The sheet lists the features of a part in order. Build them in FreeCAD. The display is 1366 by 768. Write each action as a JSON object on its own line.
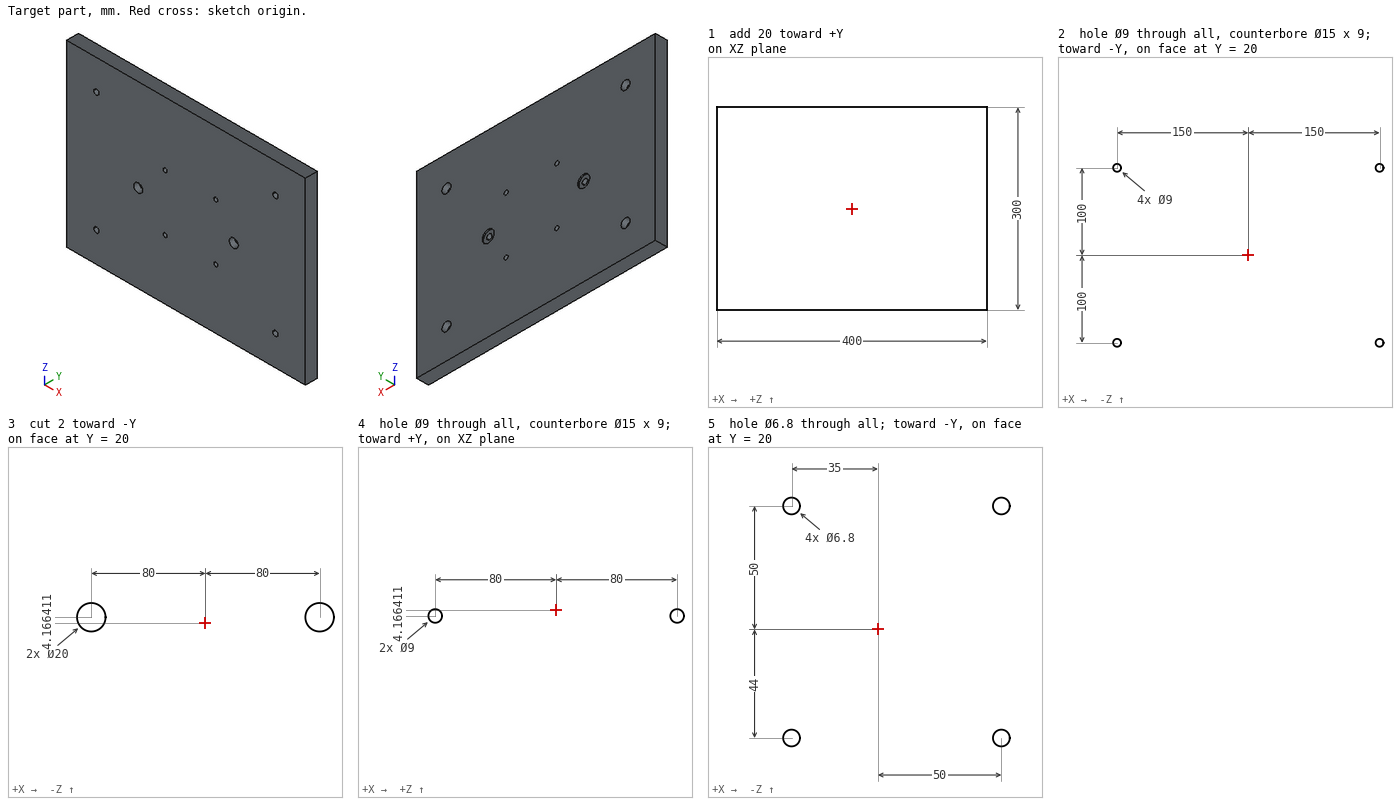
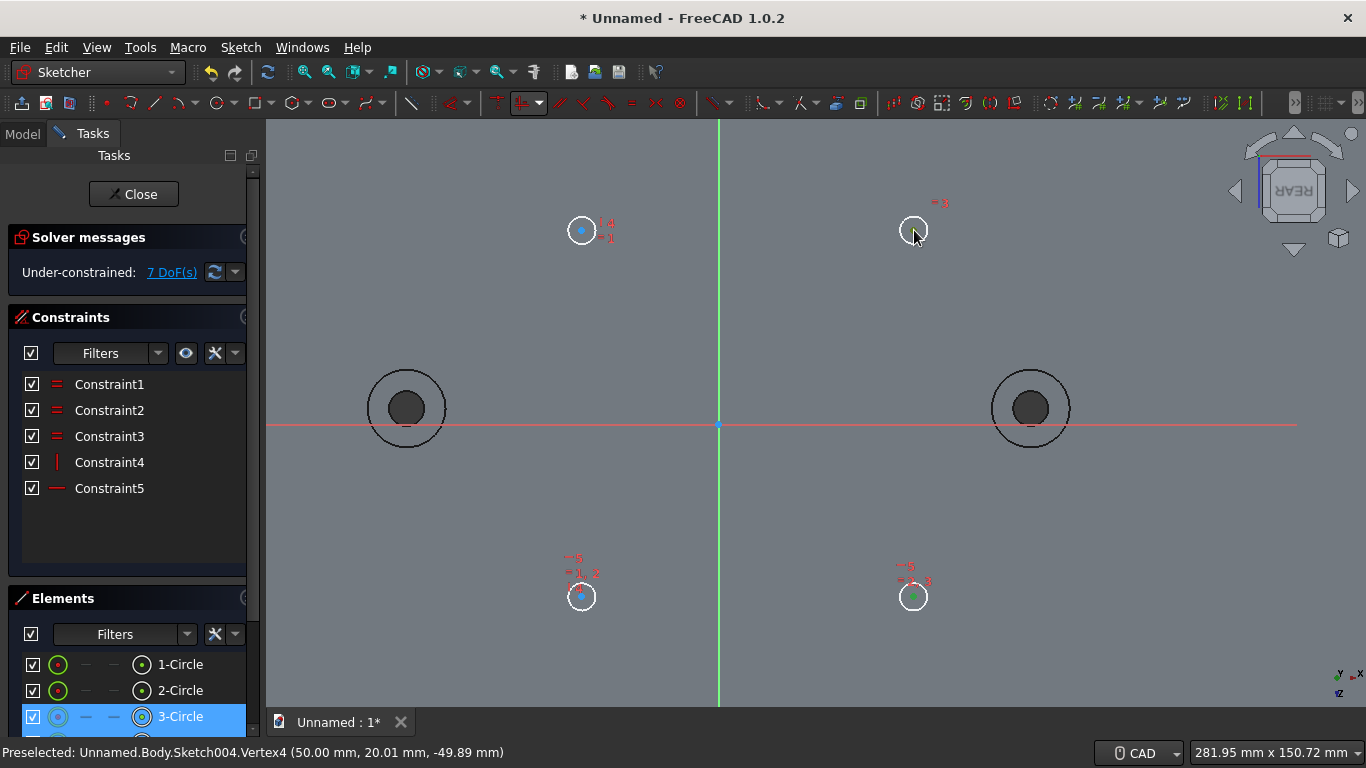
{"action": "left_click", "coordinate": [542, 104]}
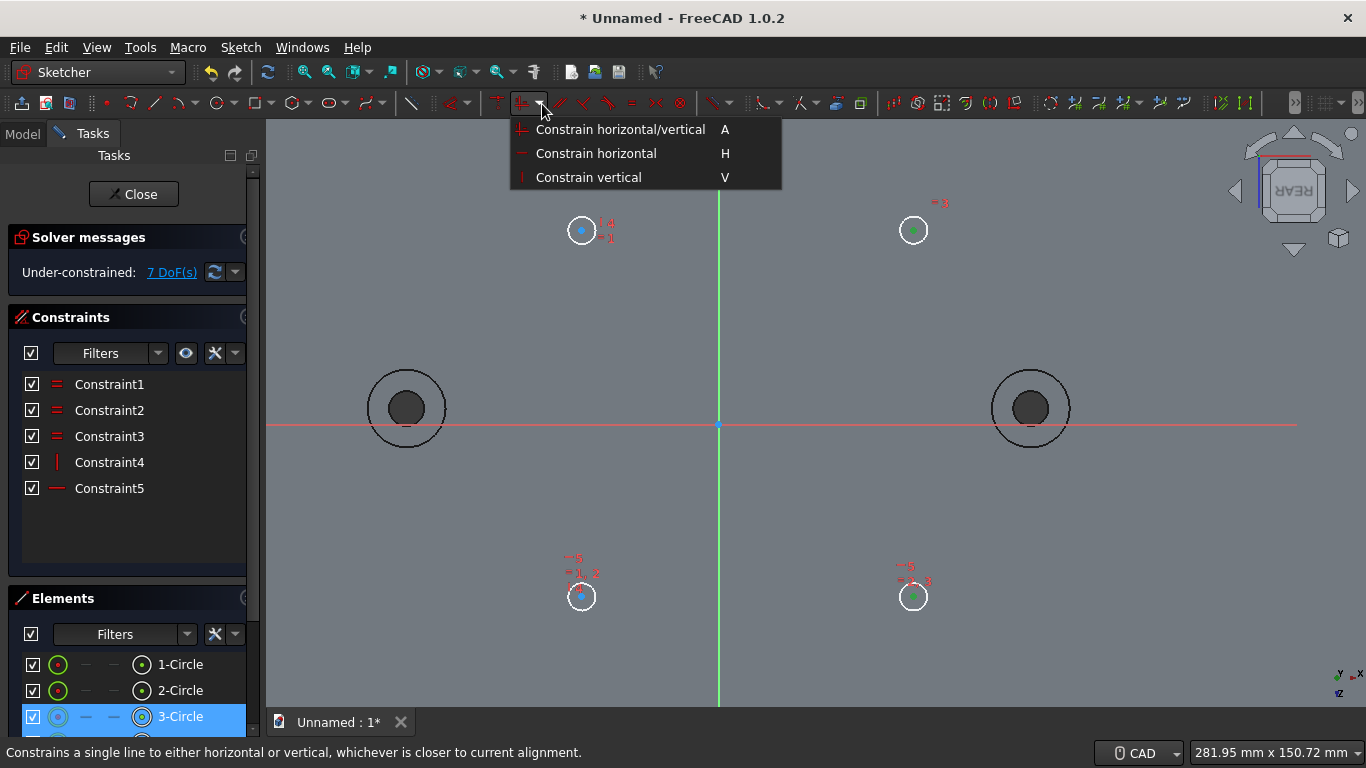
{"action": "left_click", "coordinate": [646, 177]}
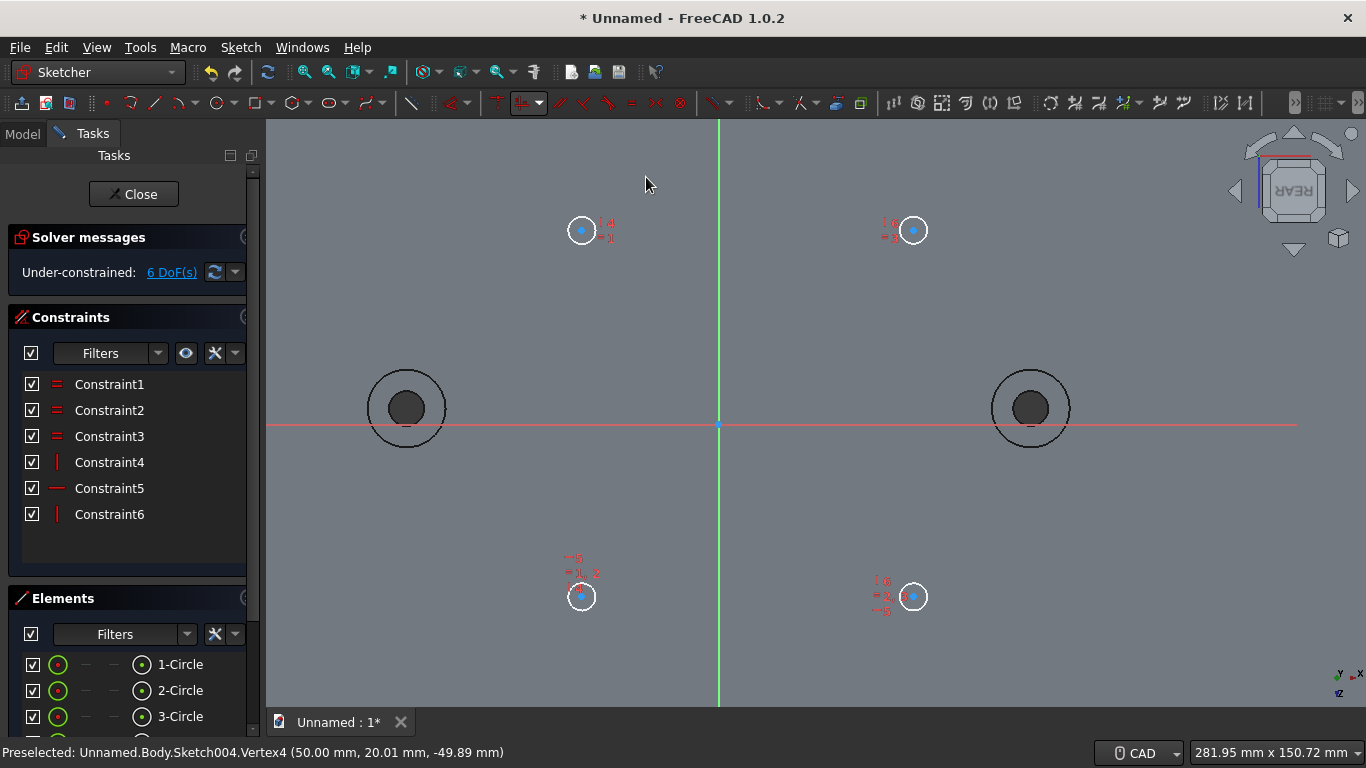
{"action": "left_click", "coordinate": [582, 231]}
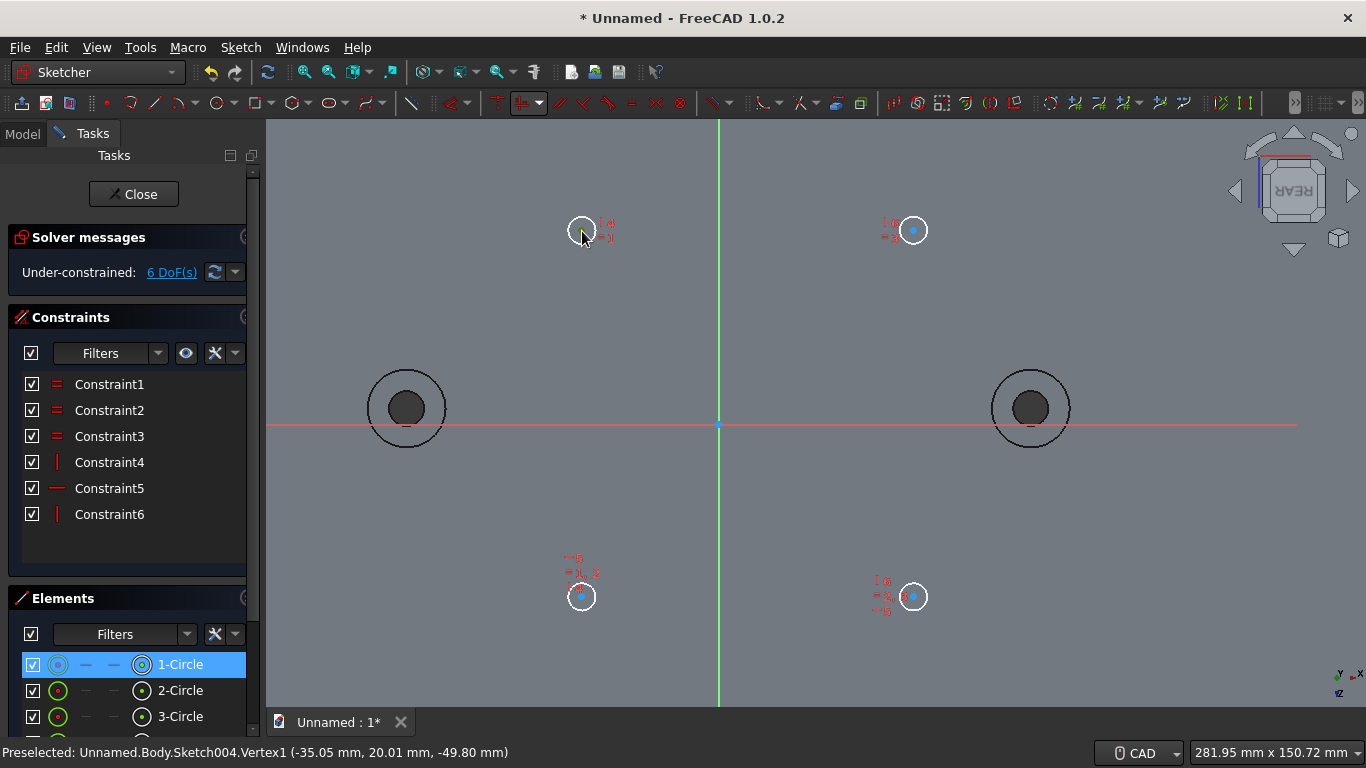
{"action": "left_click", "coordinate": [914, 230]}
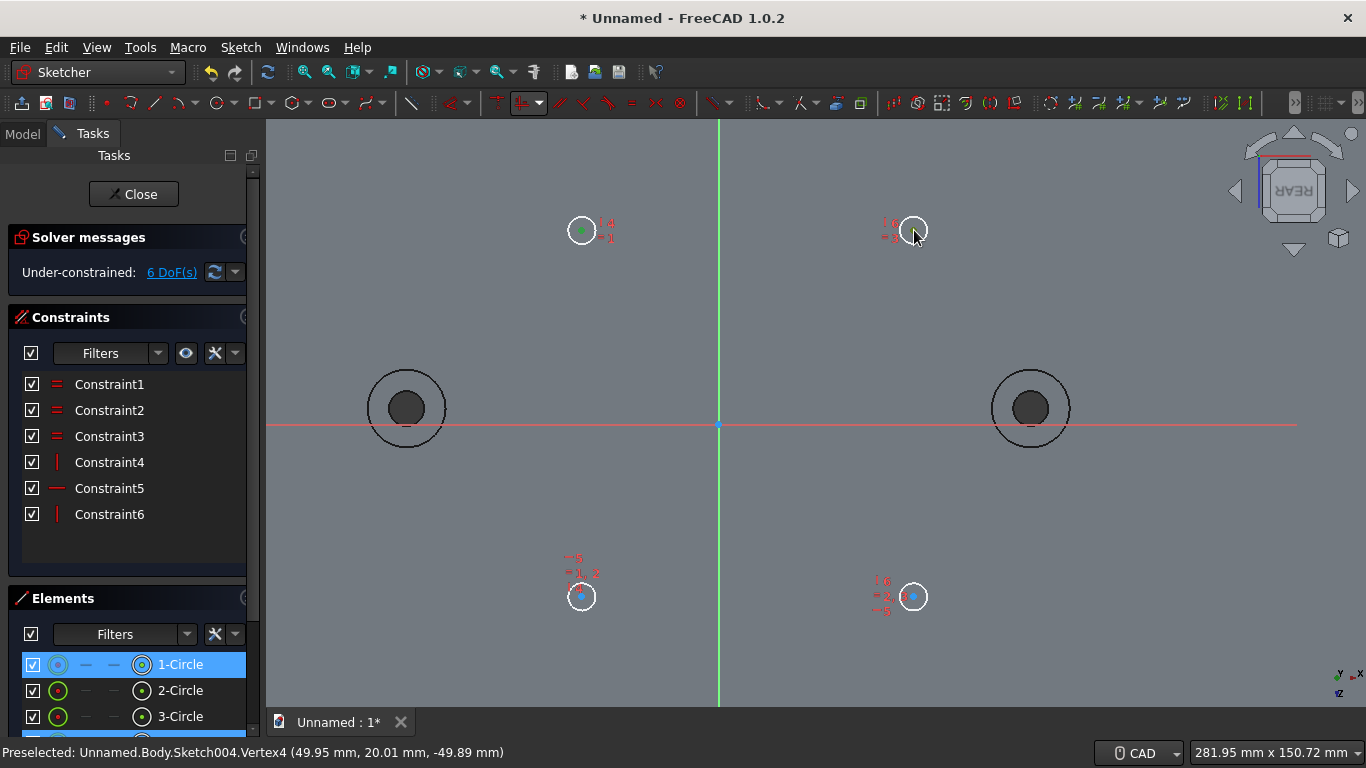
{"action": "key", "text": "h"}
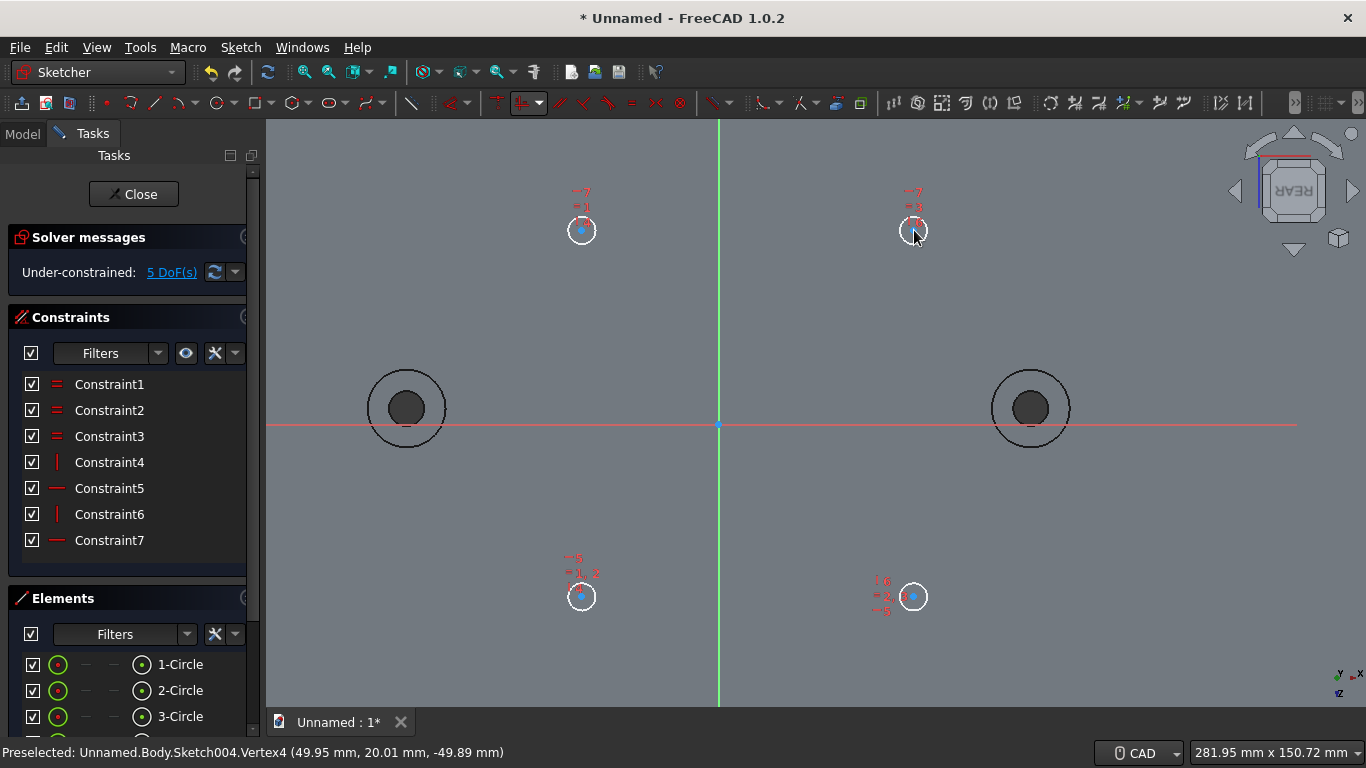
{"action": "left_click", "coordinate": [450, 104]}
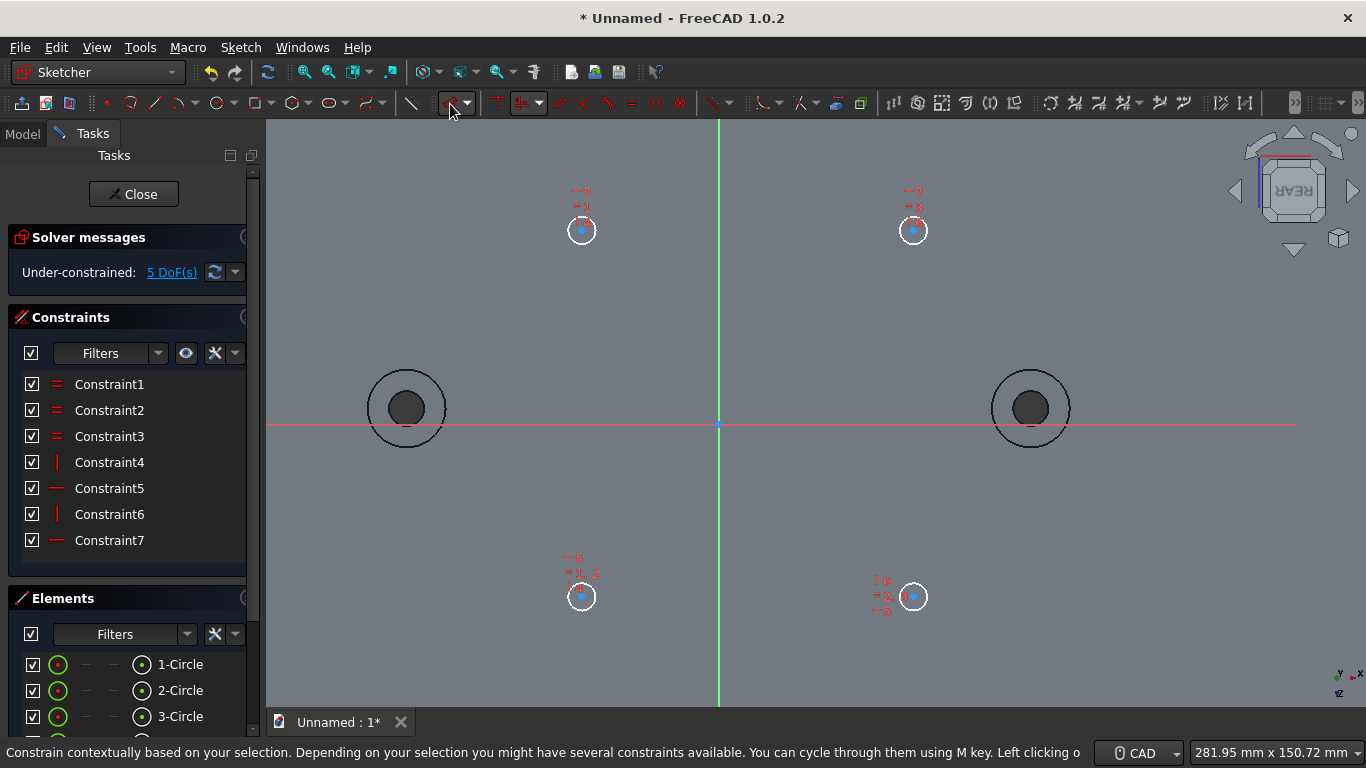
{"action": "scroll", "coordinate": [592, 221], "scroll_direction": "up", "scroll_amount": 3}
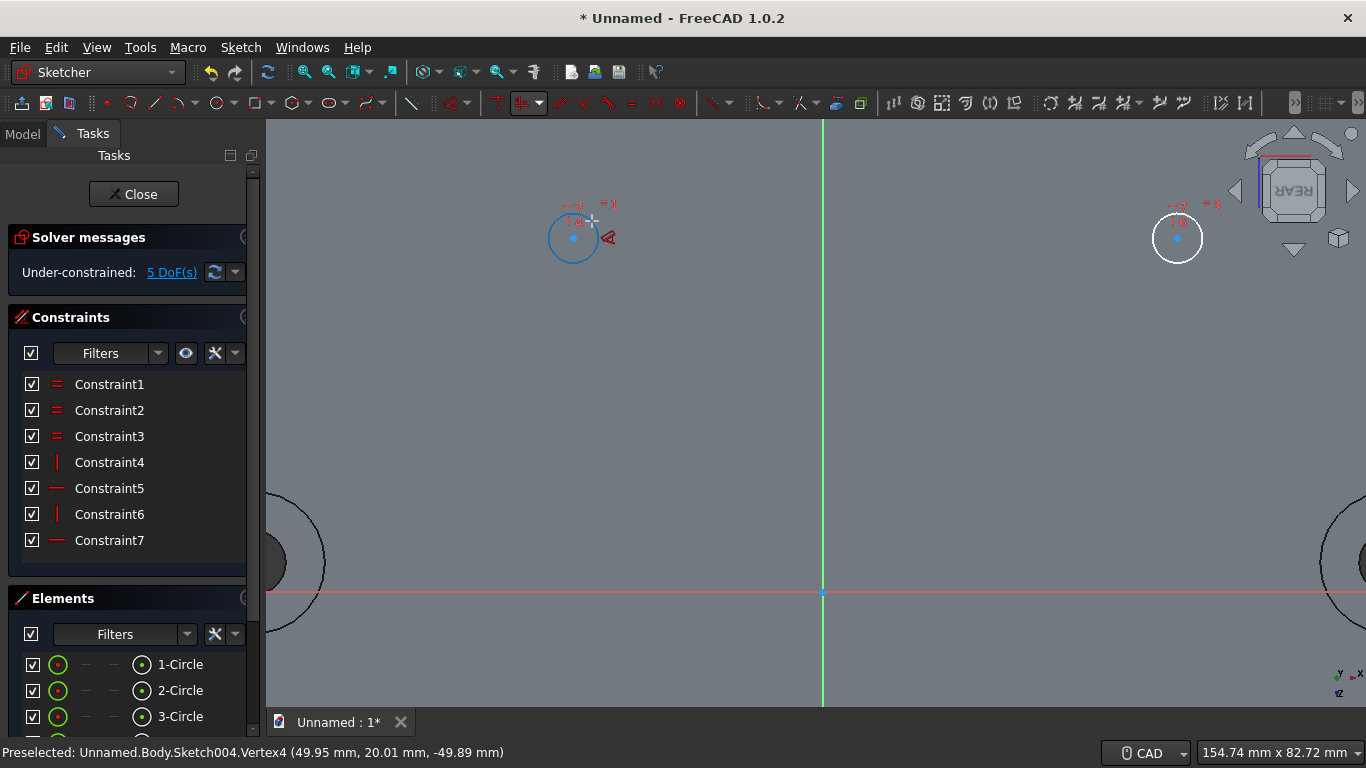
{"action": "left_click", "coordinate": [591, 221]}
{"action": "left_click", "coordinate": [614, 199]}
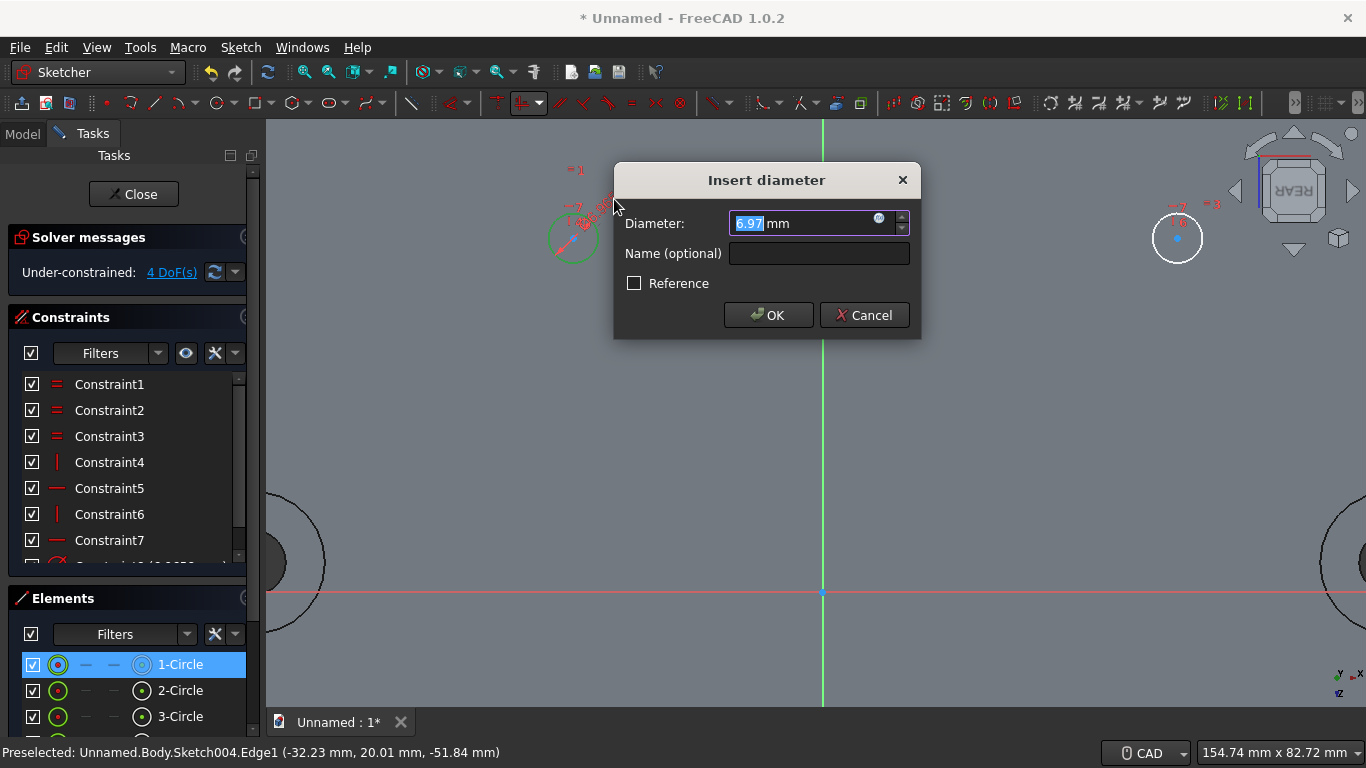
{"action": "type", "text": "6.8"}
{"action": "key", "text": "Return"}